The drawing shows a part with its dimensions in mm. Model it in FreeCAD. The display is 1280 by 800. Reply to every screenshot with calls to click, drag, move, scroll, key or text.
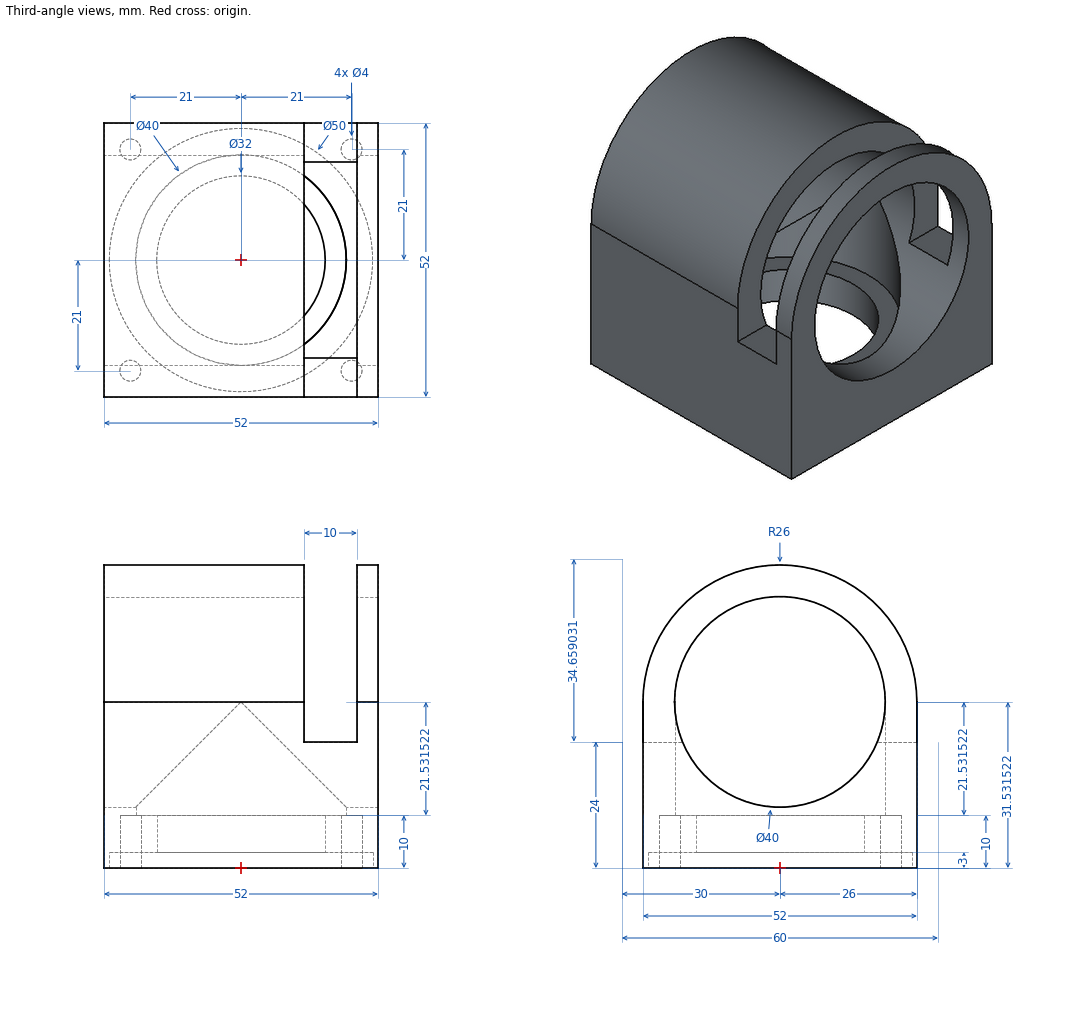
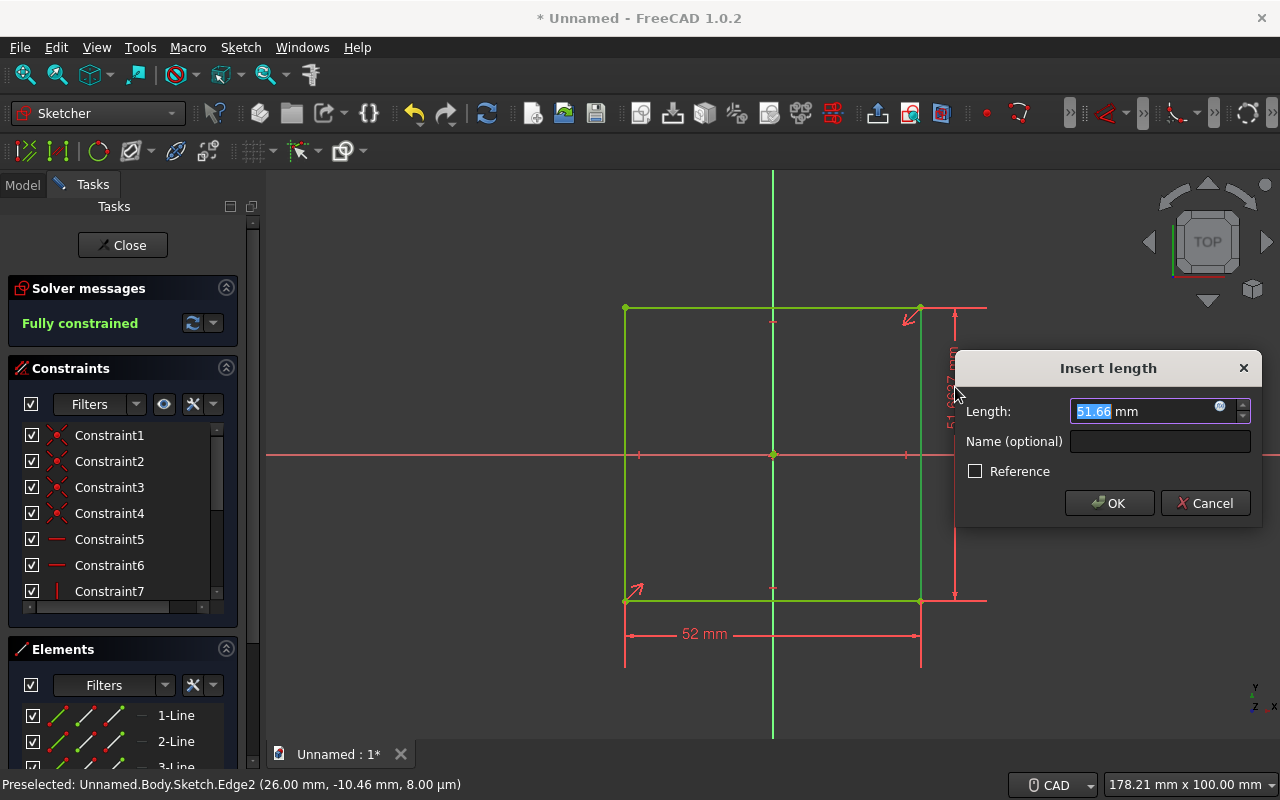
text(52)
key(Return)
key(Escape)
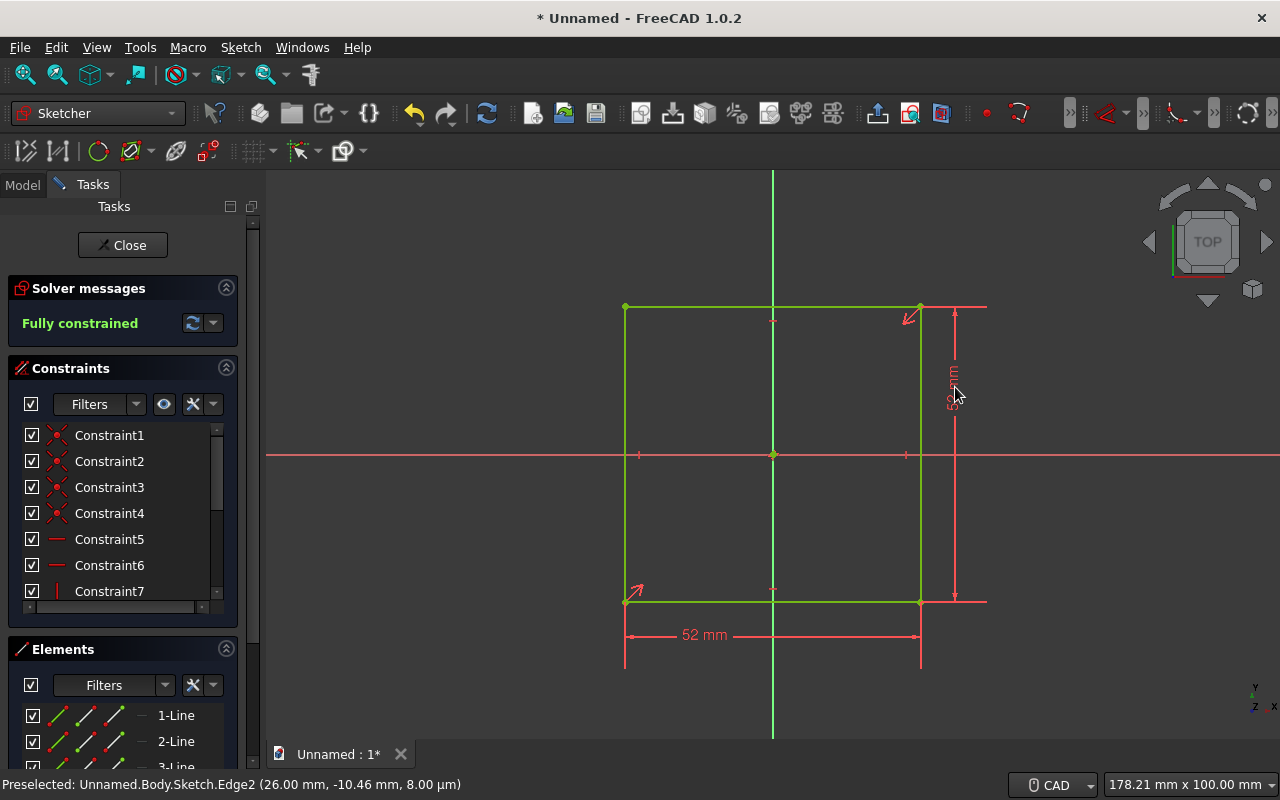
click(123, 245)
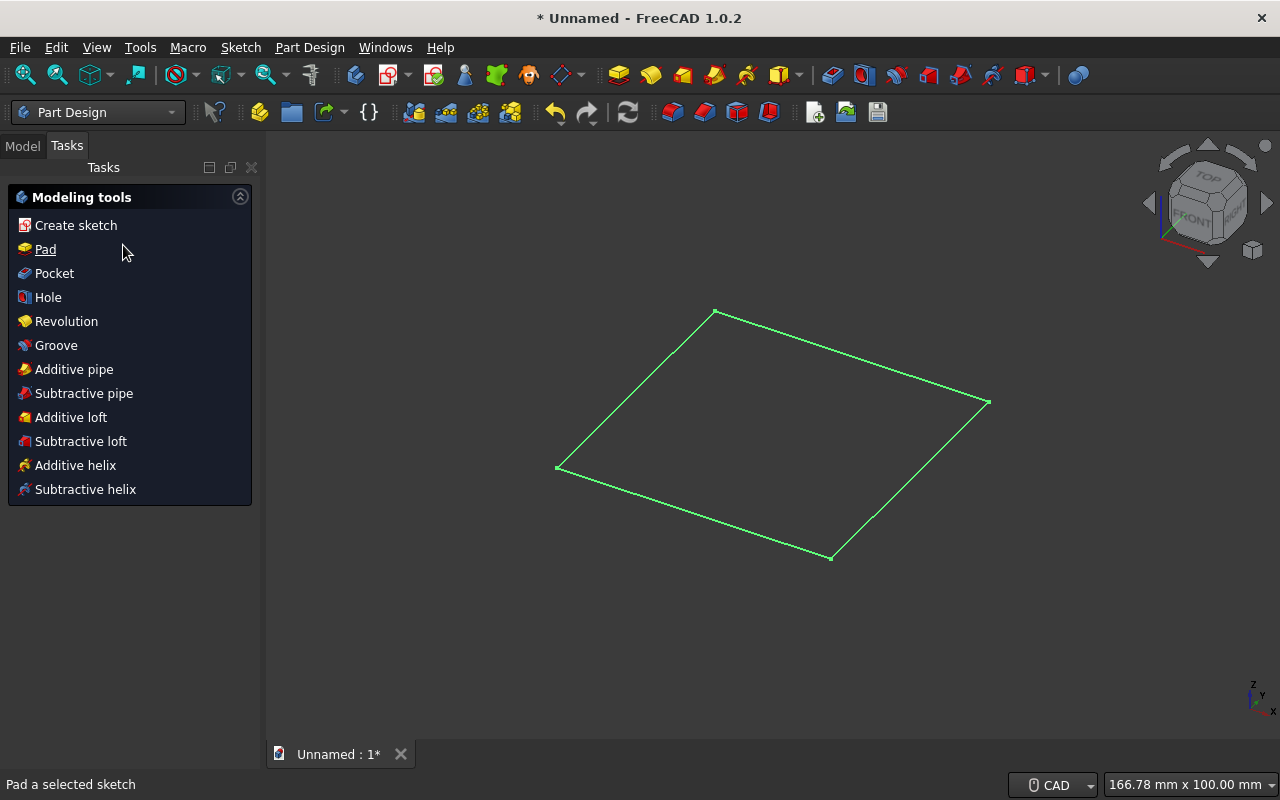
click(620, 76)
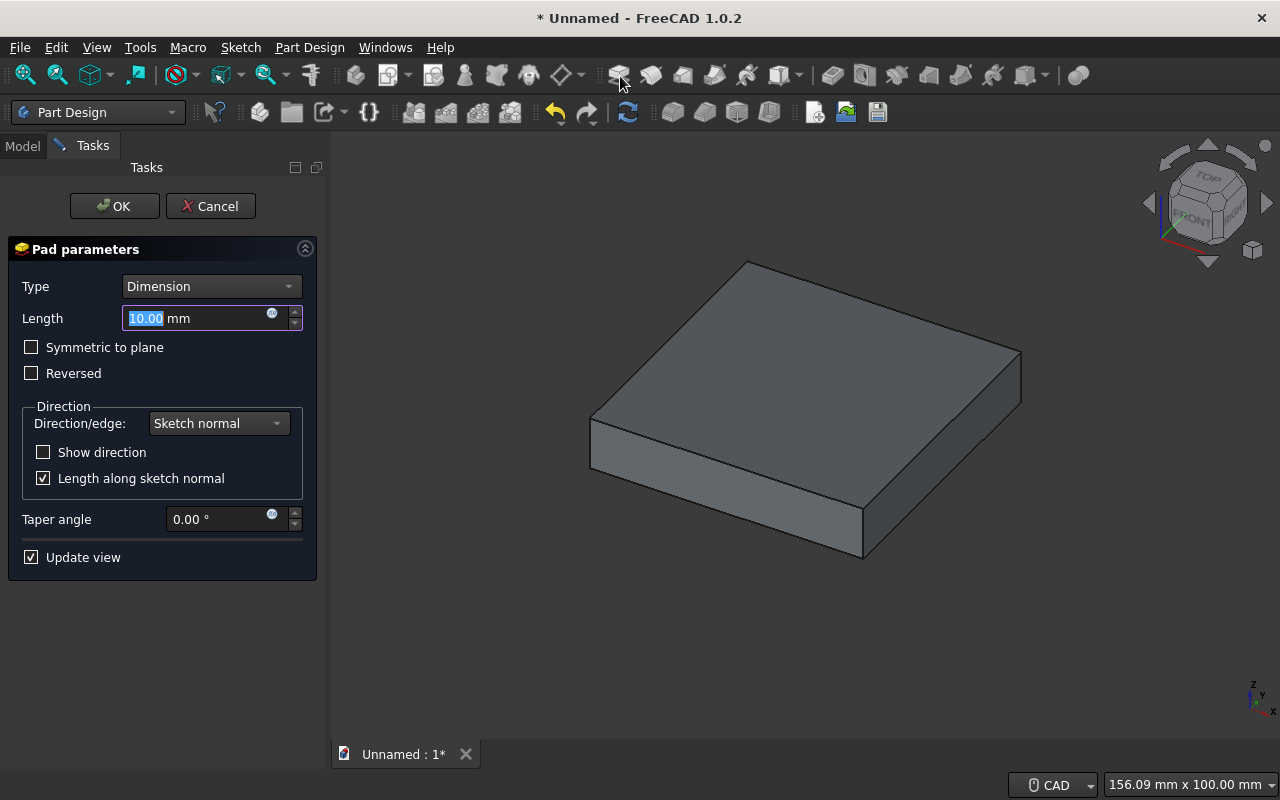
text(10)
key(Tab)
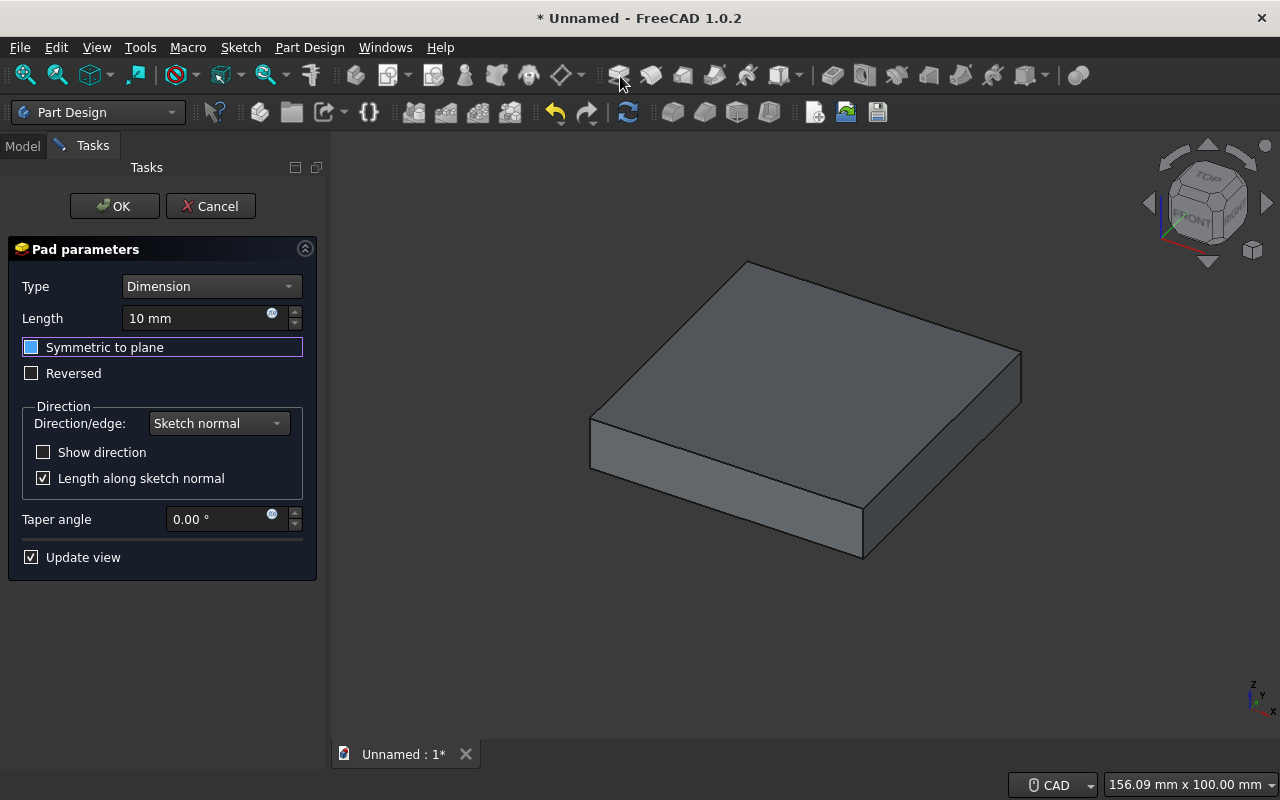
click(115, 206)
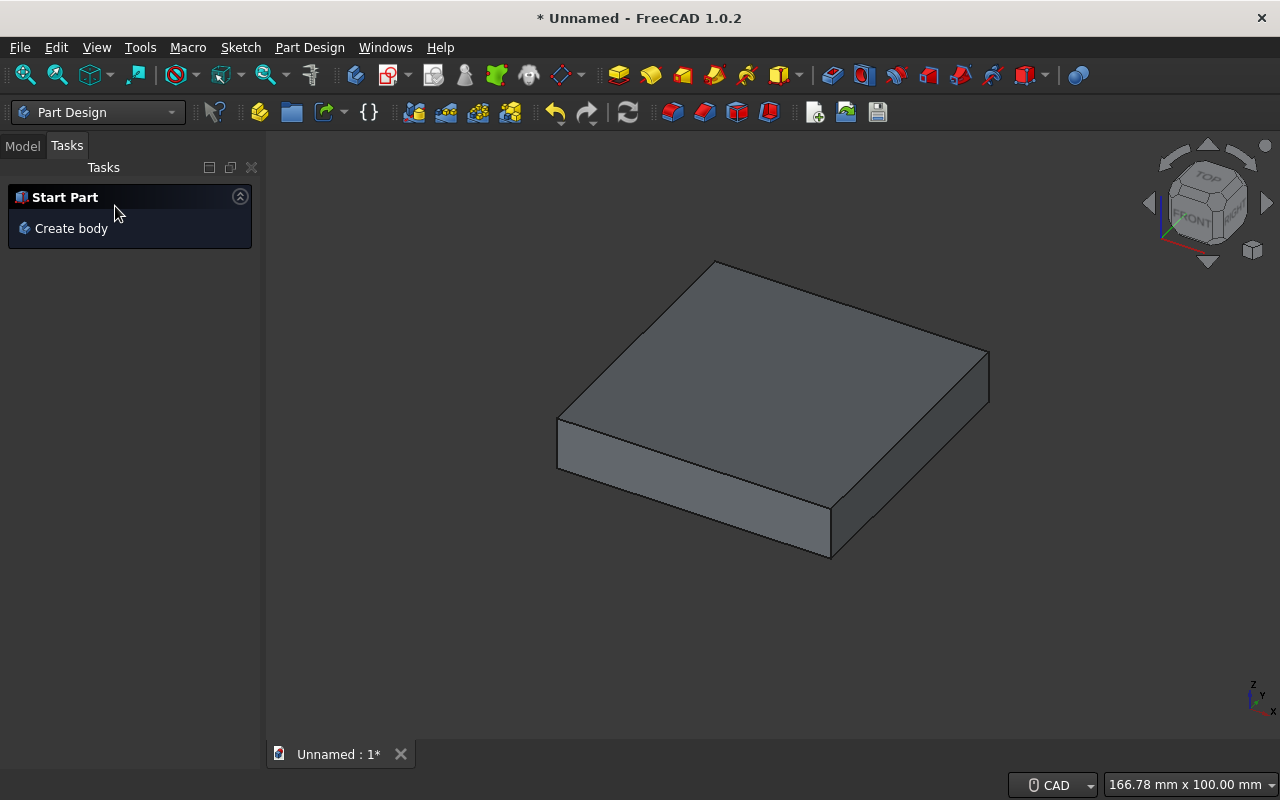
click(388, 76)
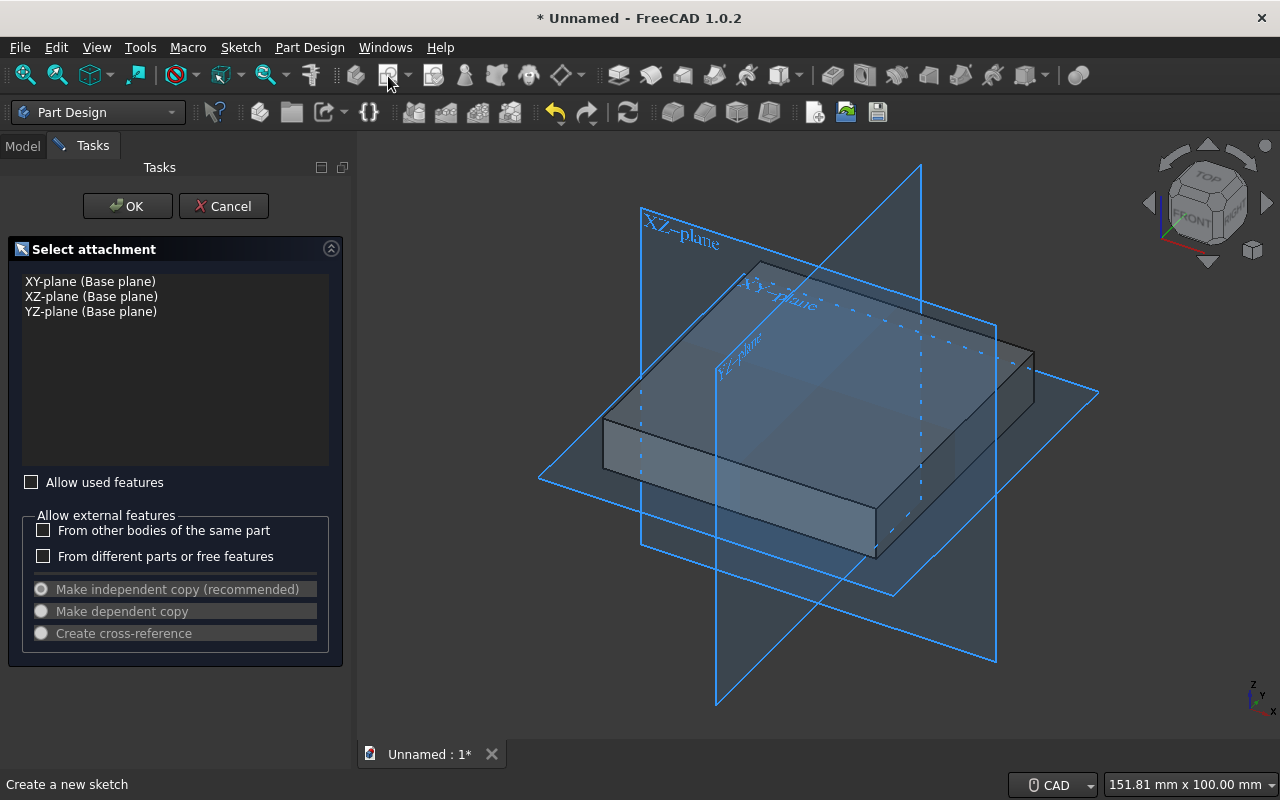
click(82, 282)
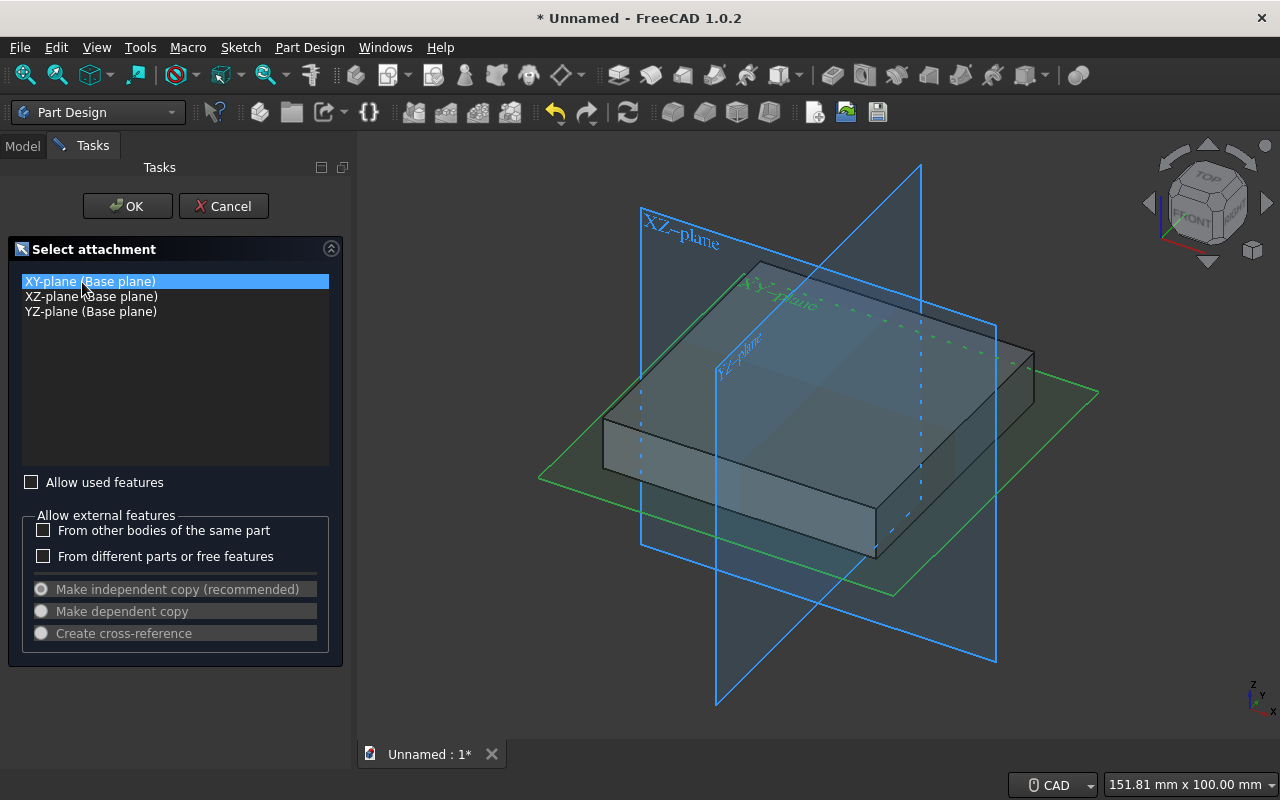
click(128, 206)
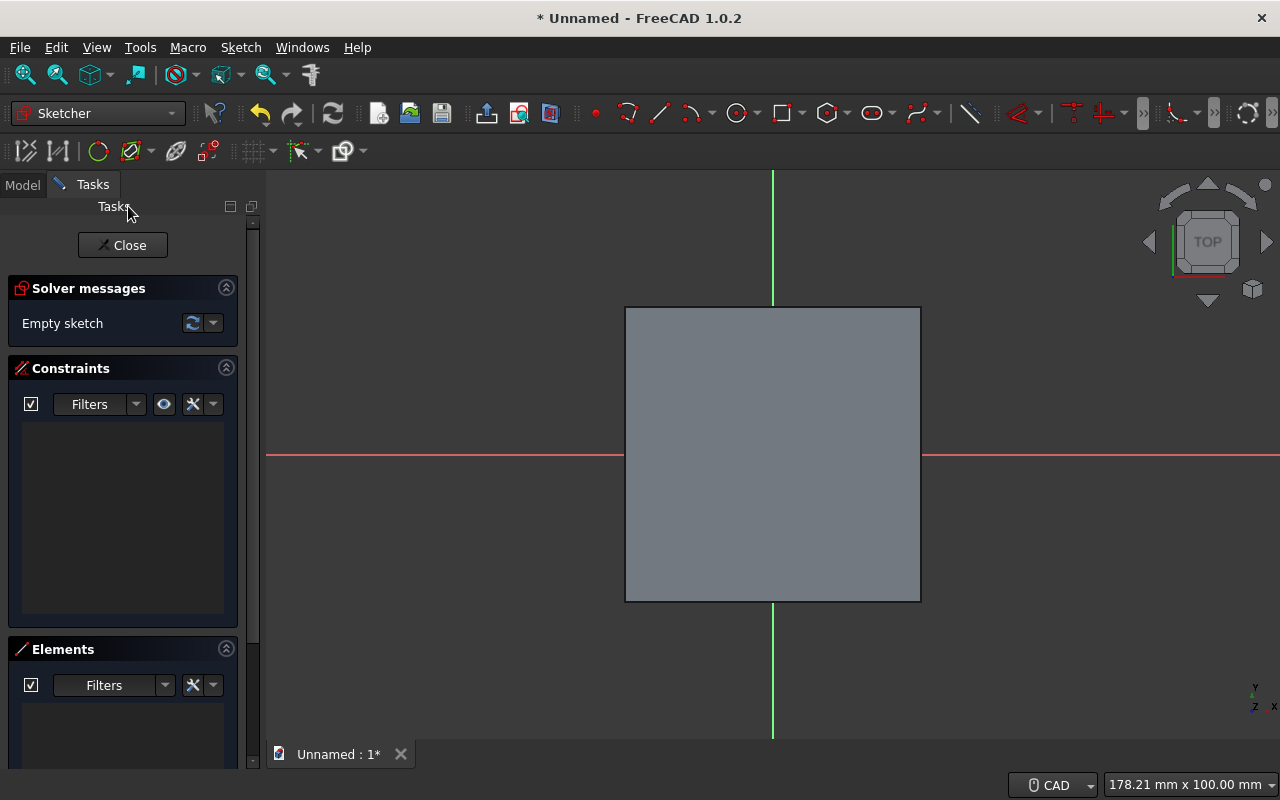
click(552, 114)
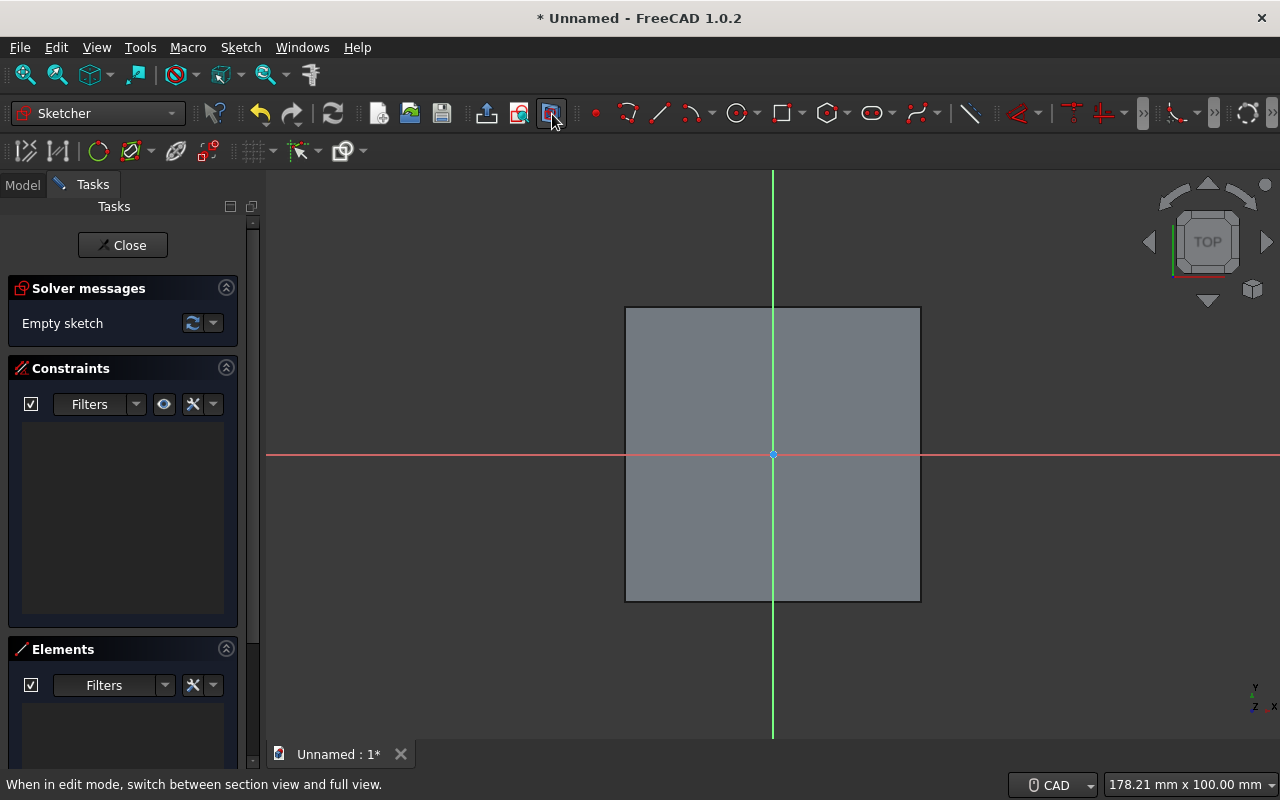
scroll(912, 455, up, 2)